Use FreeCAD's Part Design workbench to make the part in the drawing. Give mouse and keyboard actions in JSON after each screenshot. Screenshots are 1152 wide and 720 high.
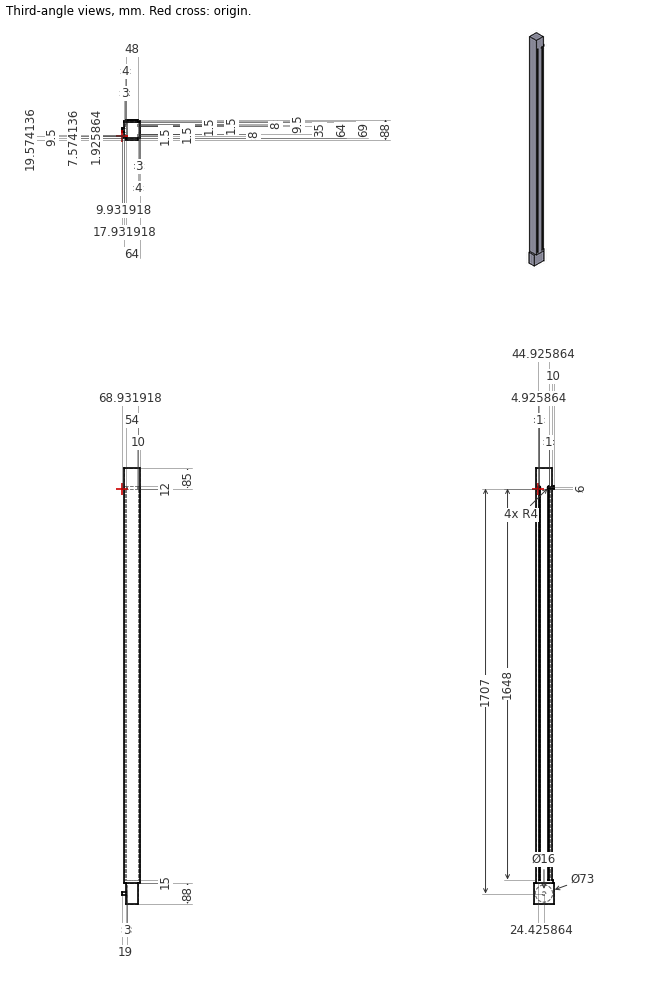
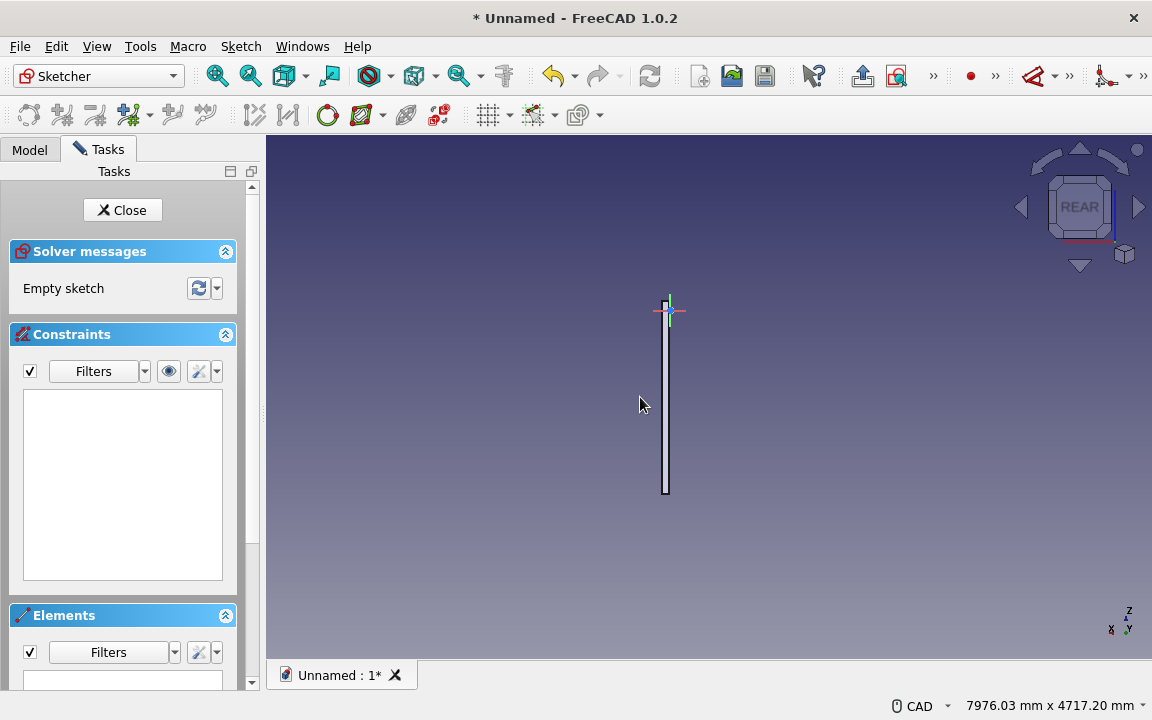
{"action": "scroll", "coordinate": [668, 305], "scroll_direction": "up", "scroll_amount": 15}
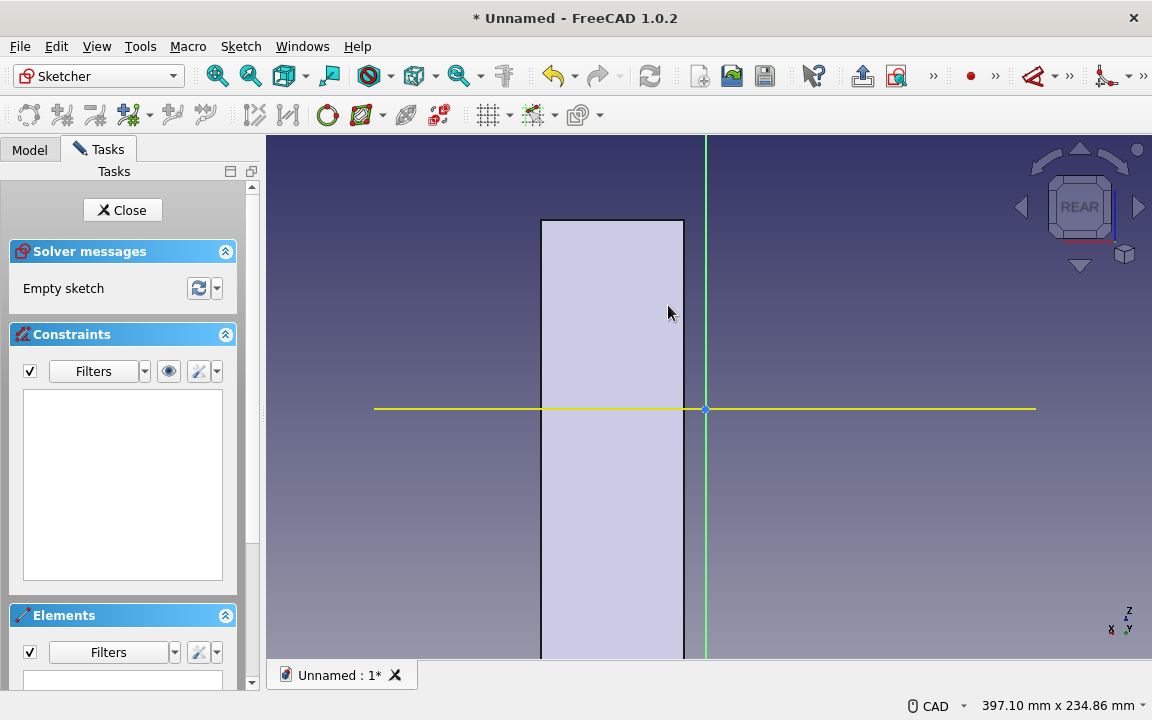
{"action": "scroll", "coordinate": [624, 396], "scroll_direction": "up", "scroll_amount": 6}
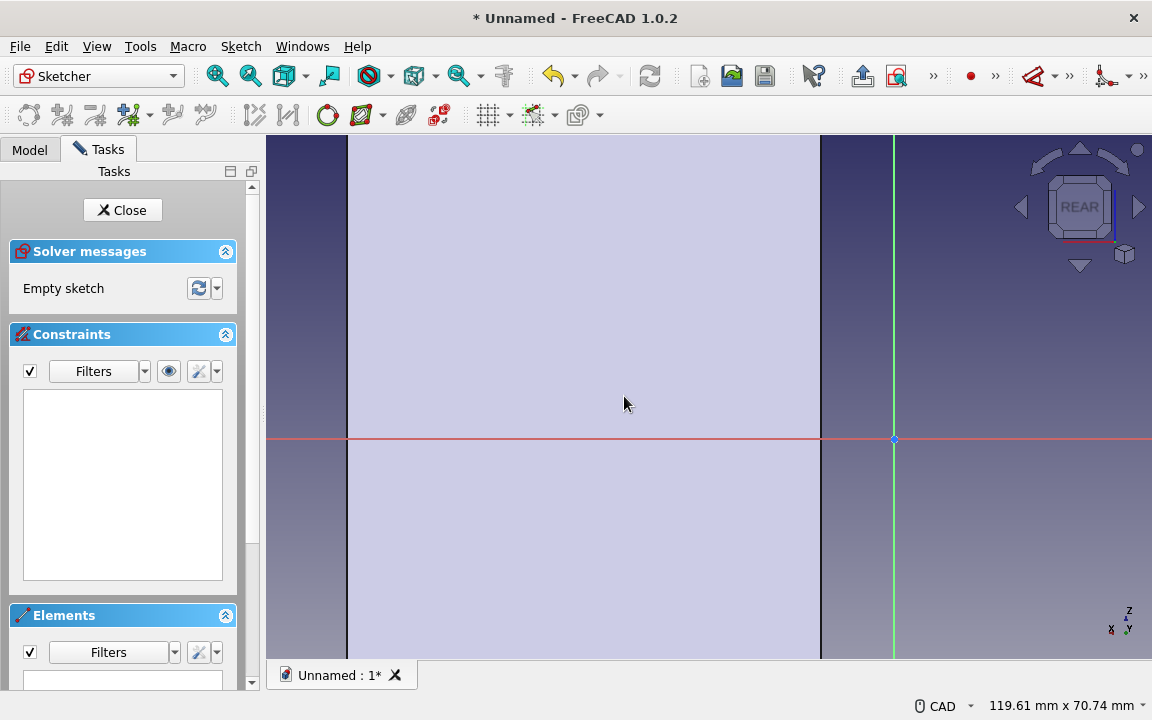
{"action": "key", "text": "g r"}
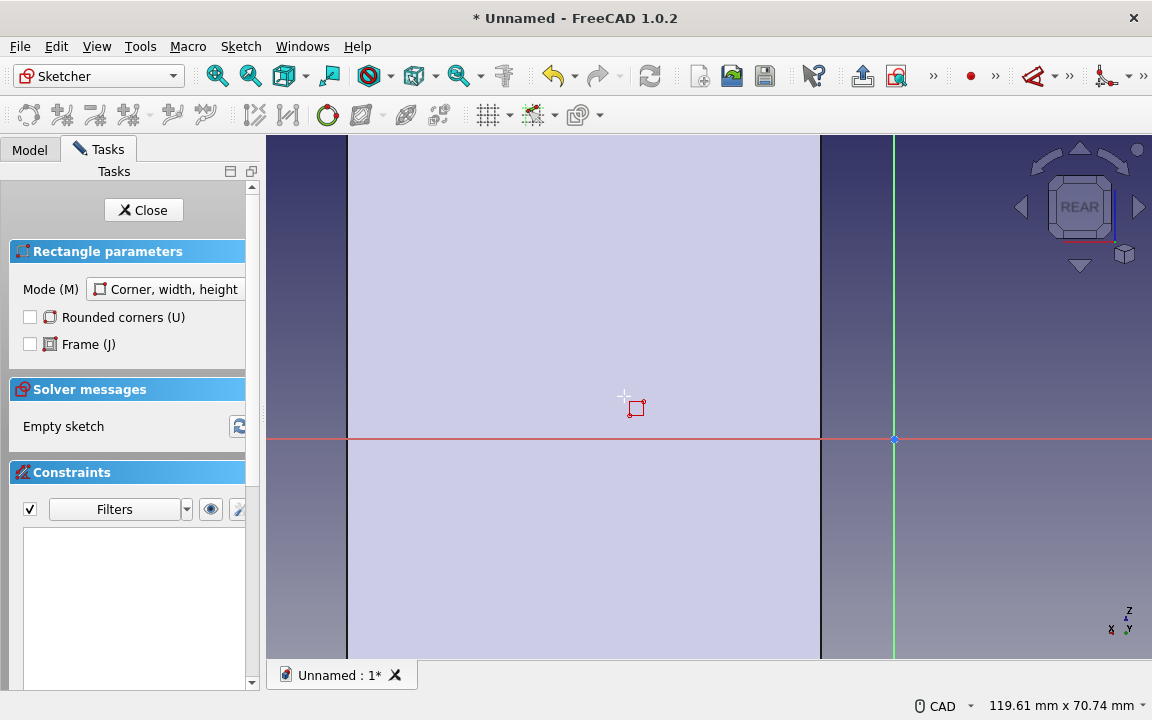
{"action": "left_click", "coordinate": [384, 350]}
{"action": "left_click", "coordinate": [784, 439]}
{"action": "key", "text": "Escape"}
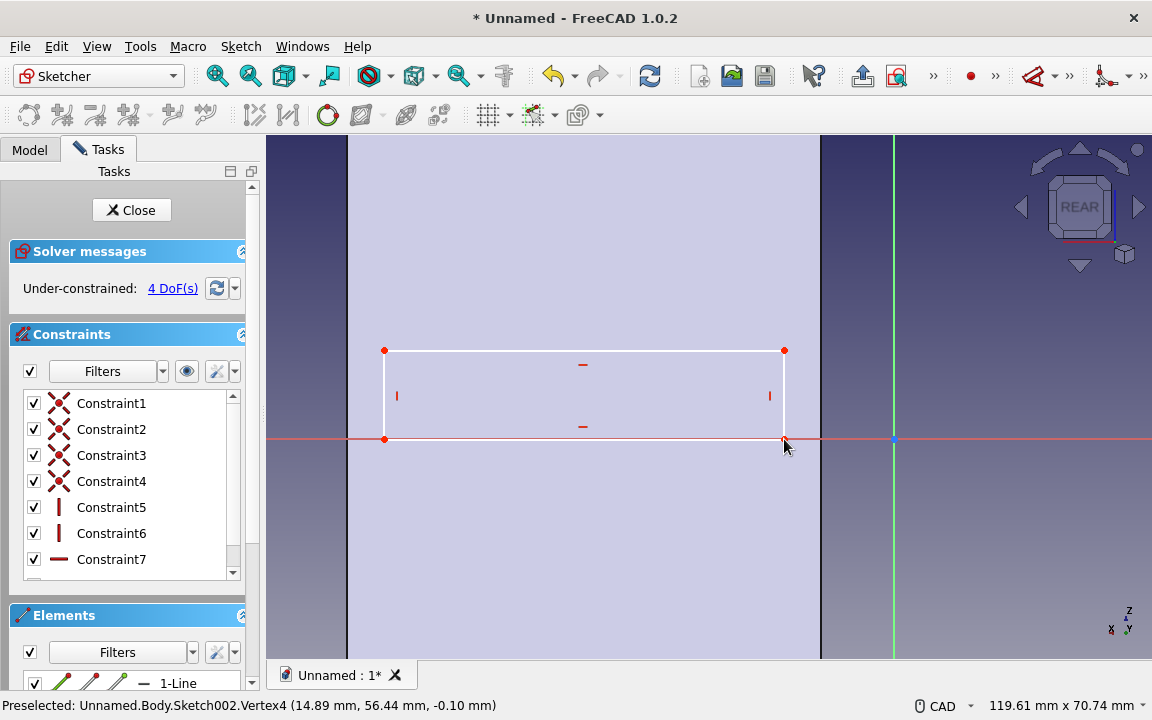
{"action": "left_click", "coordinate": [384, 440]}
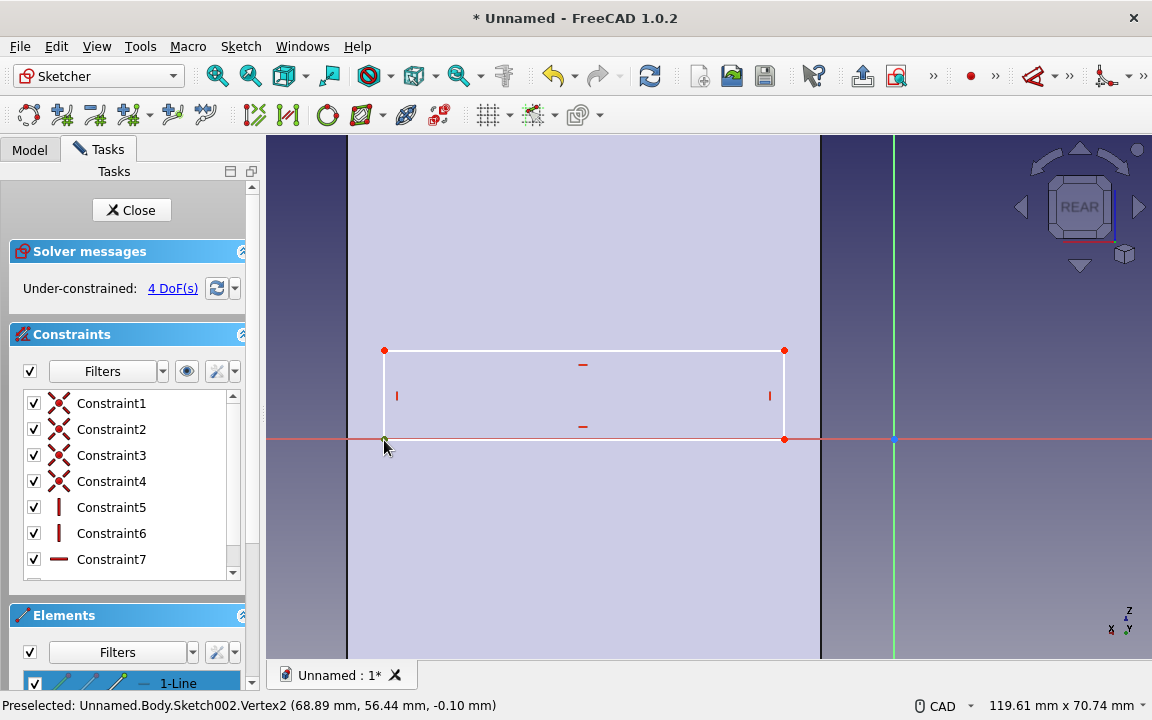
{"action": "left_click", "coordinate": [344, 439]}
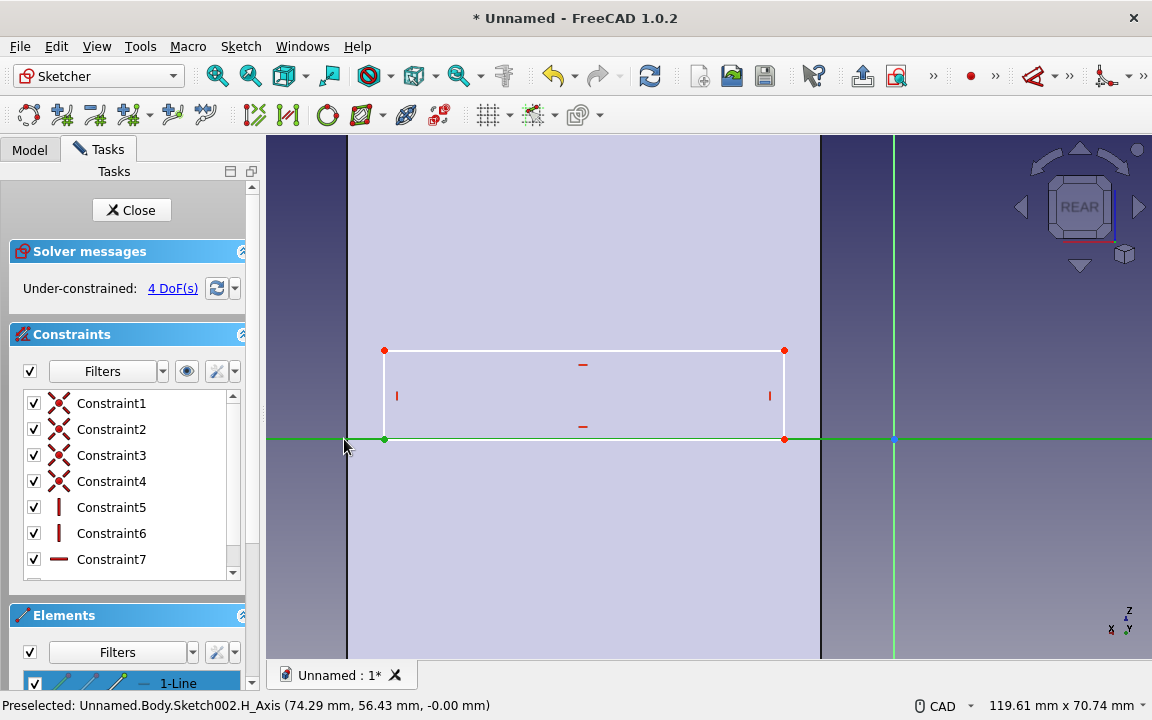
{"action": "key", "text": "c"}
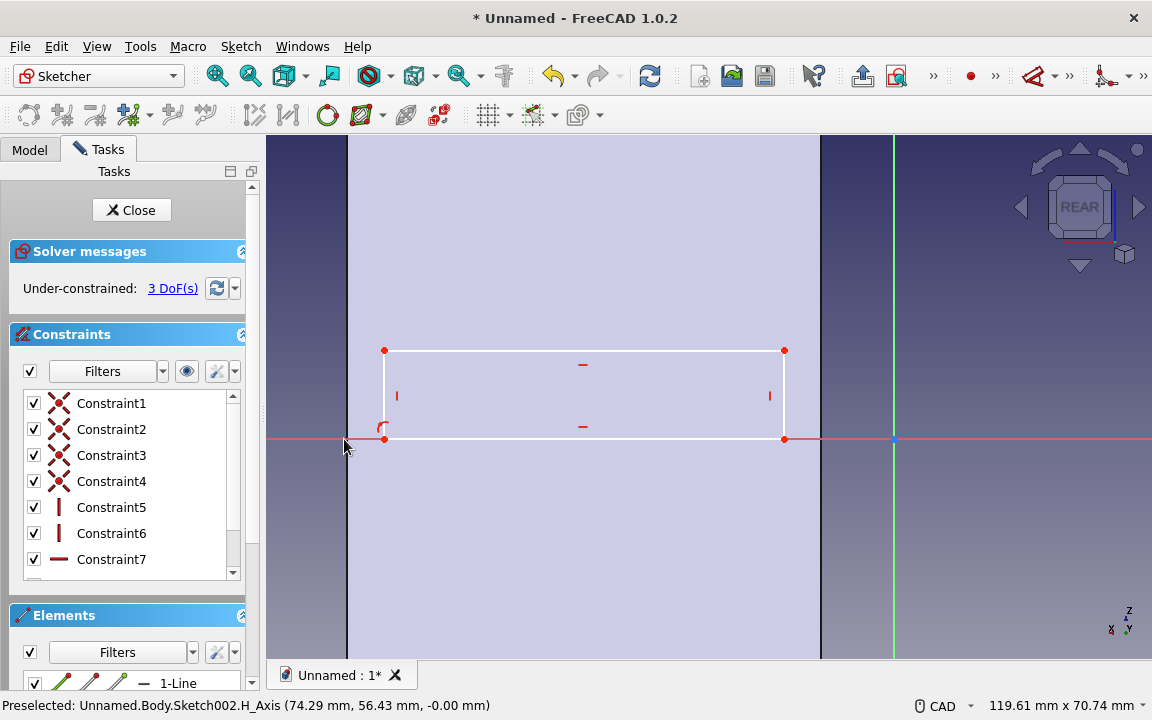
{"action": "left_click", "coordinate": [1032, 76]}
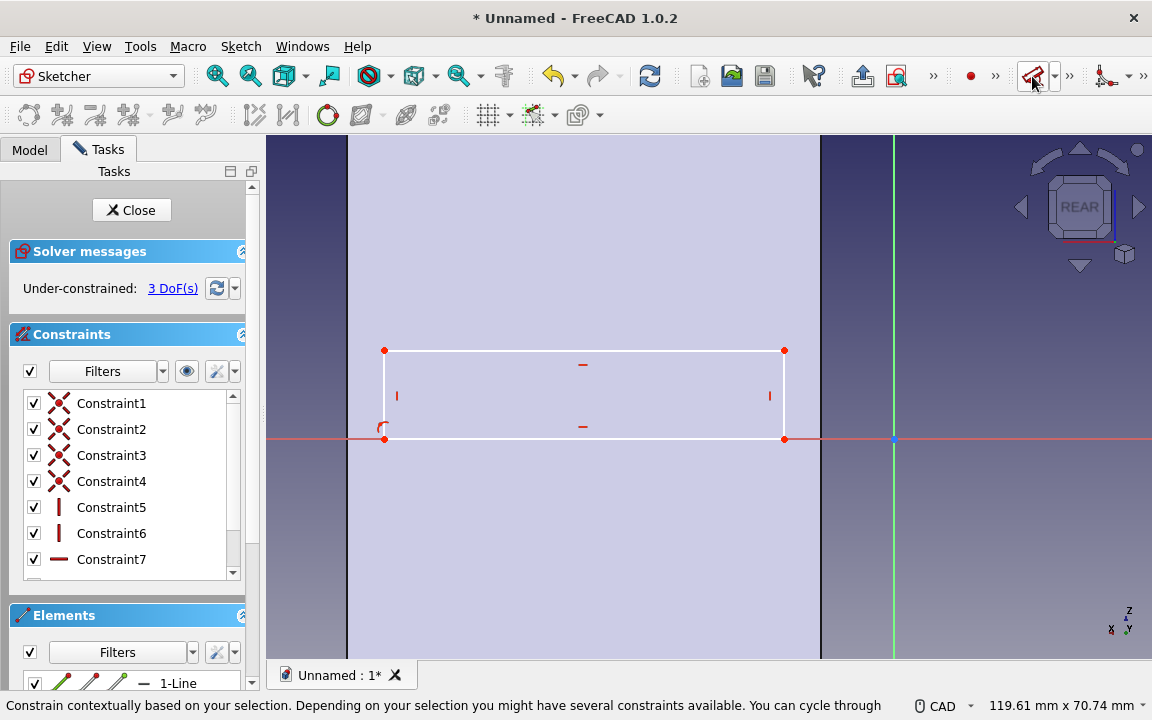
{"action": "left_click", "coordinate": [384, 377]}
{"action": "left_click", "coordinate": [350, 395]}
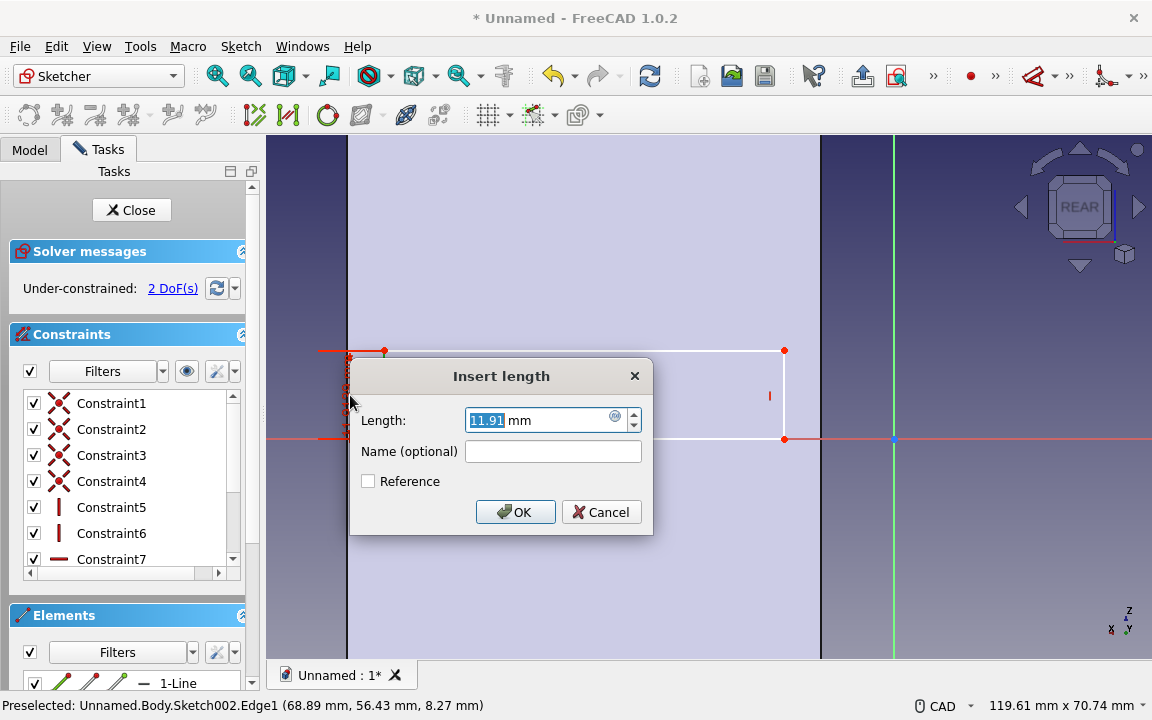
{"action": "type", "text": "12"}
{"action": "key", "text": "Return"}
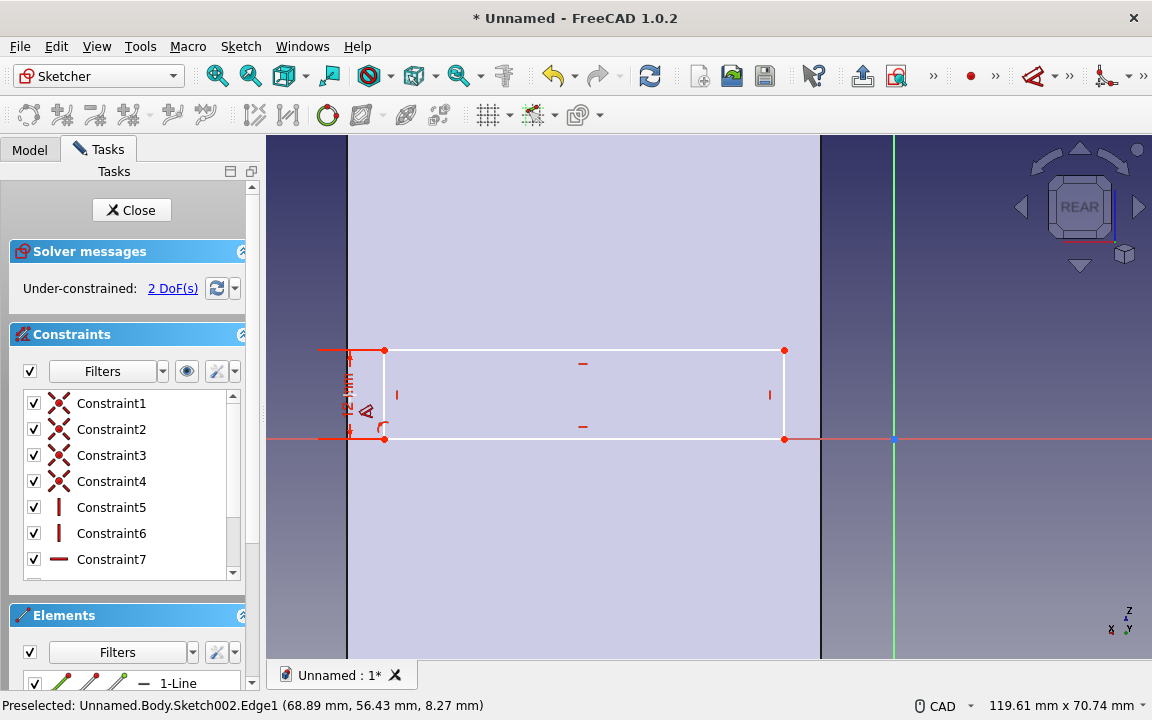
{"action": "left_click", "coordinate": [504, 439]}
{"action": "left_click", "coordinate": [584, 473]}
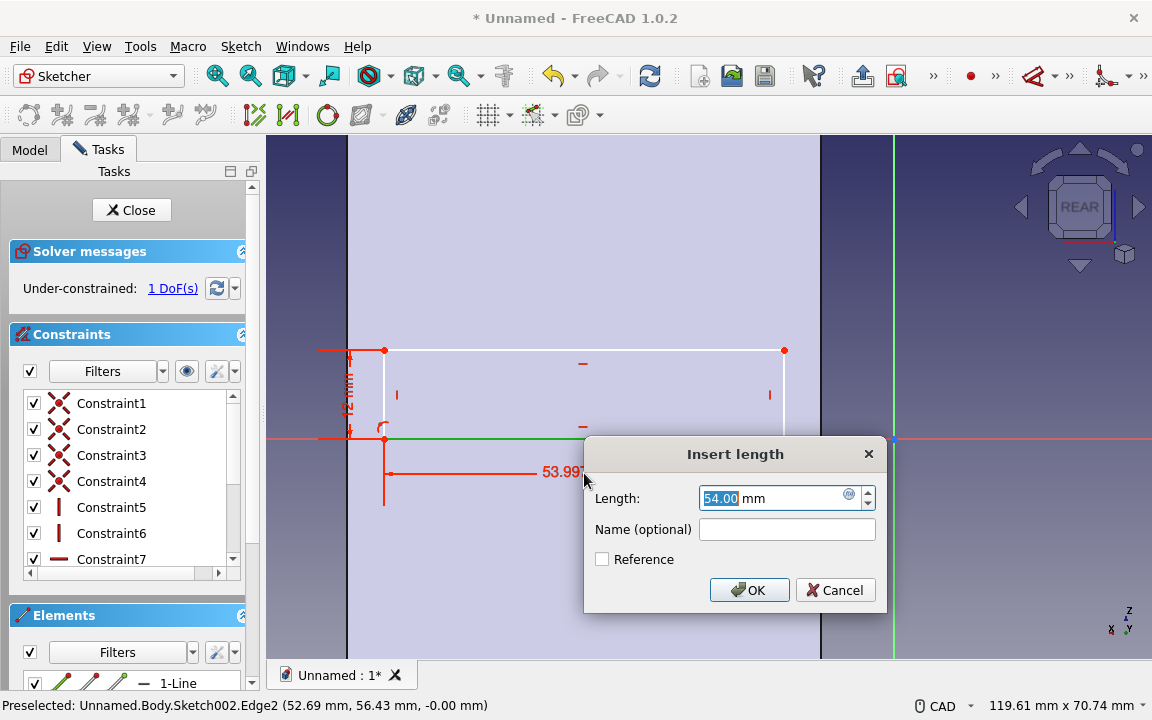
{"action": "type", "text": "54"}
{"action": "key", "text": "Return"}